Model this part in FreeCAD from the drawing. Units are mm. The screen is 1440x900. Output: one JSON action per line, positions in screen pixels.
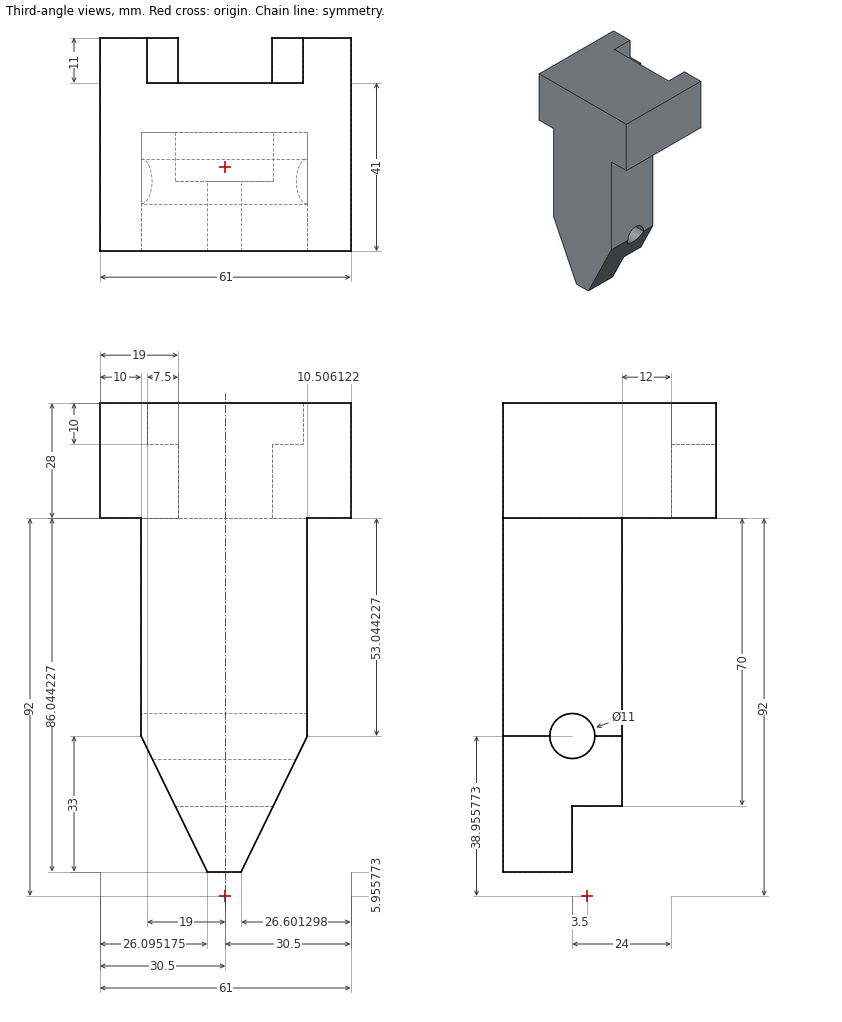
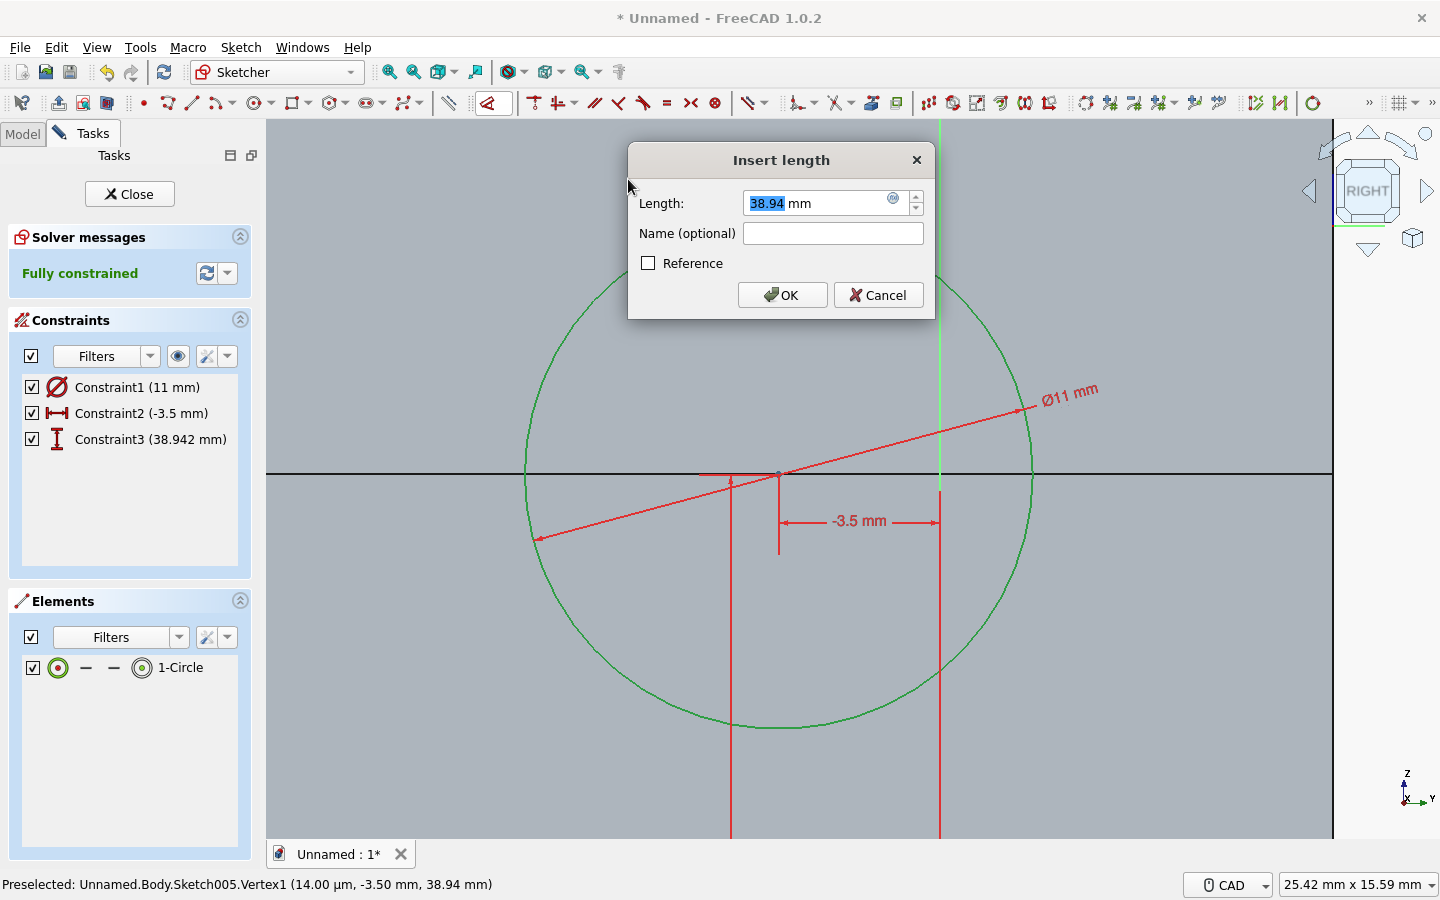
{"action": "type", "text": "38.955773"}
{"action": "key", "text": "Return"}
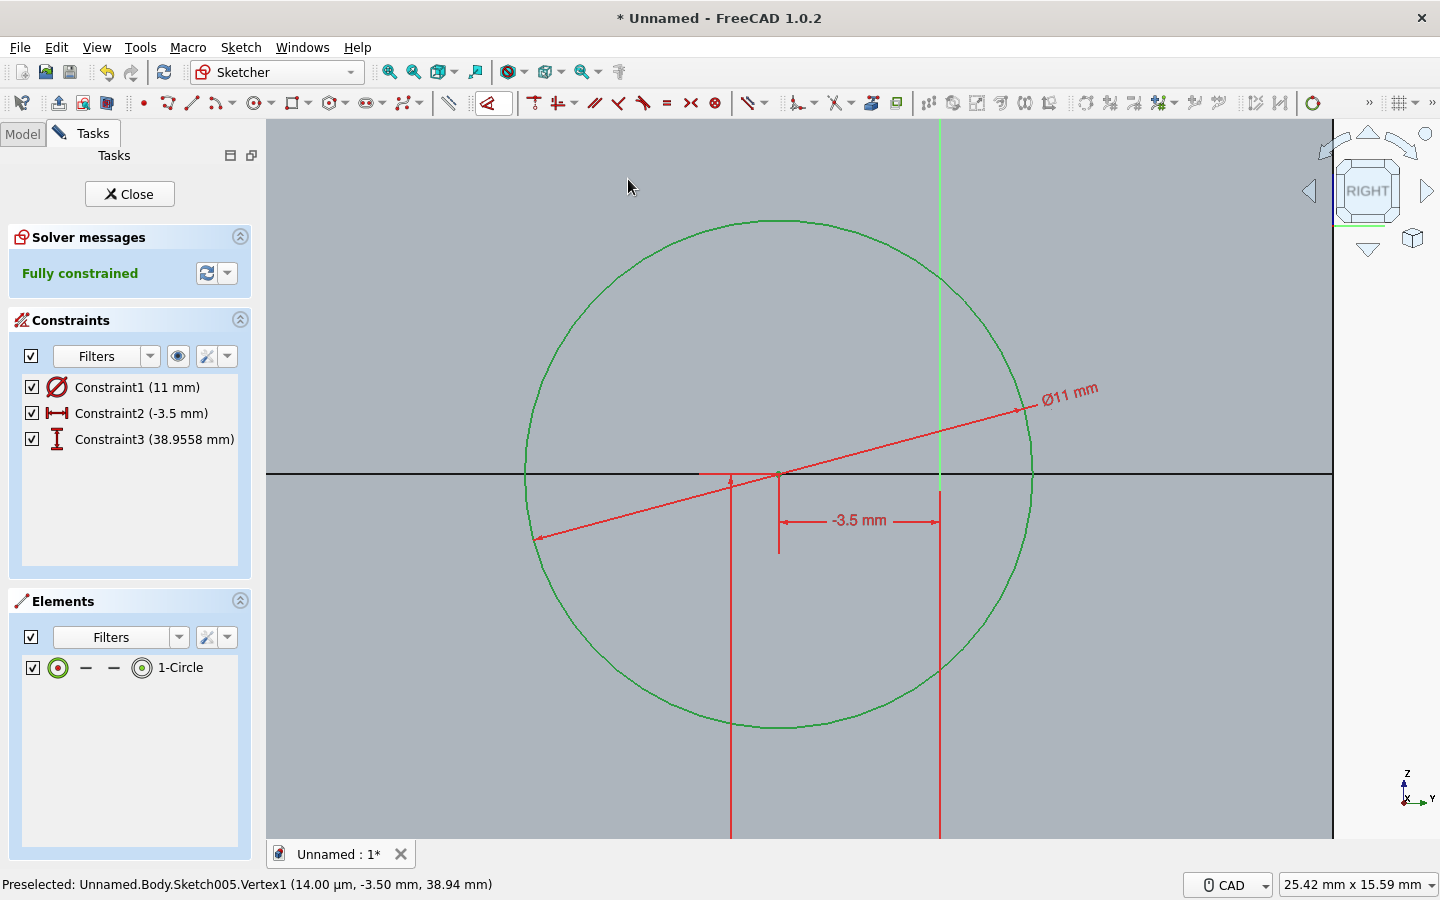
{"action": "left_click", "coordinate": [130, 194]}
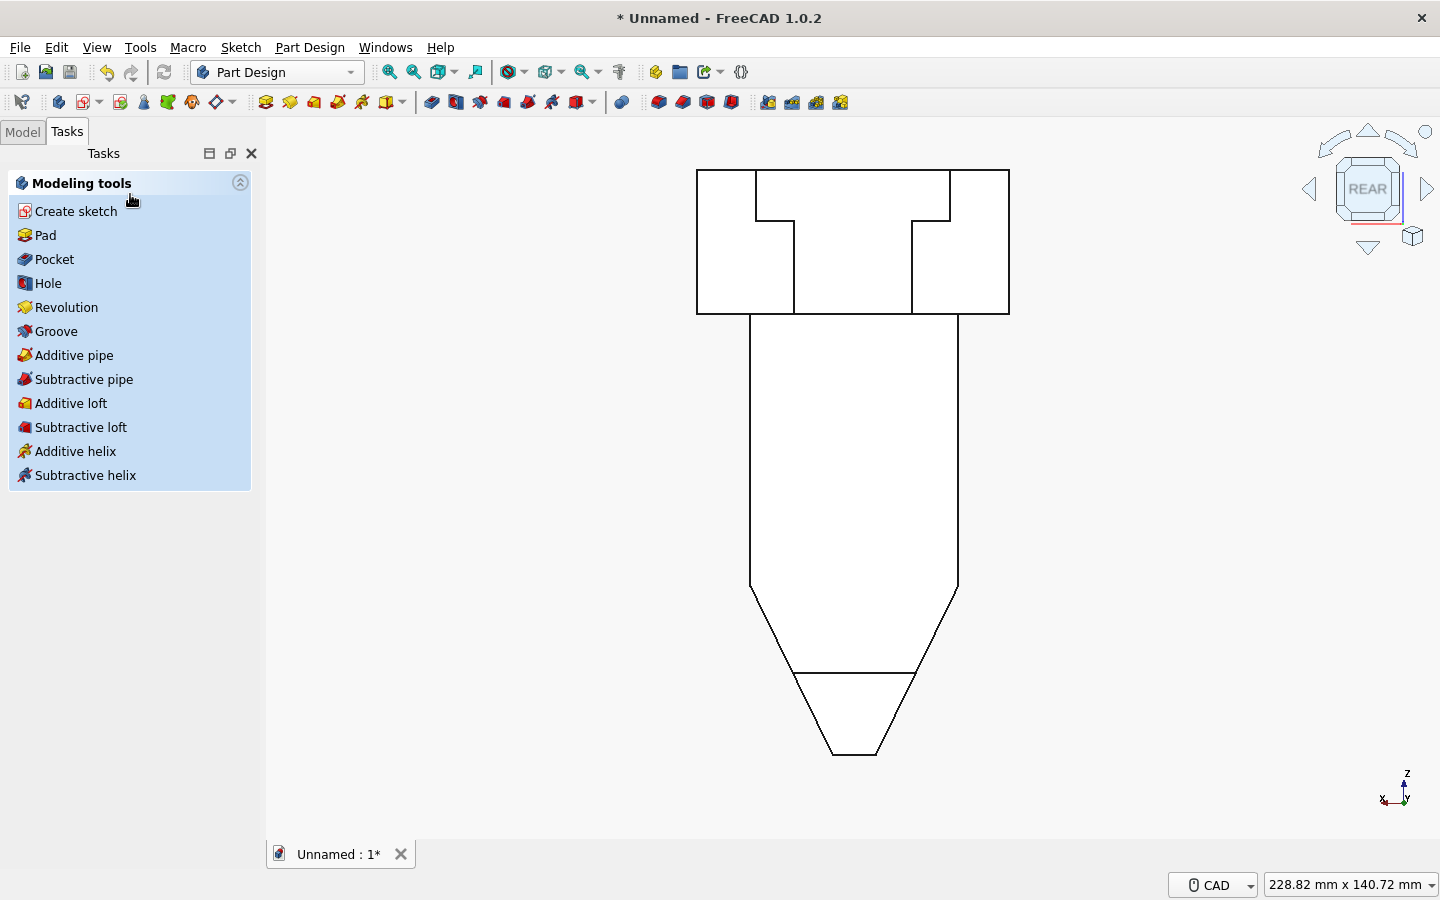
{"action": "left_click", "coordinate": [432, 102]}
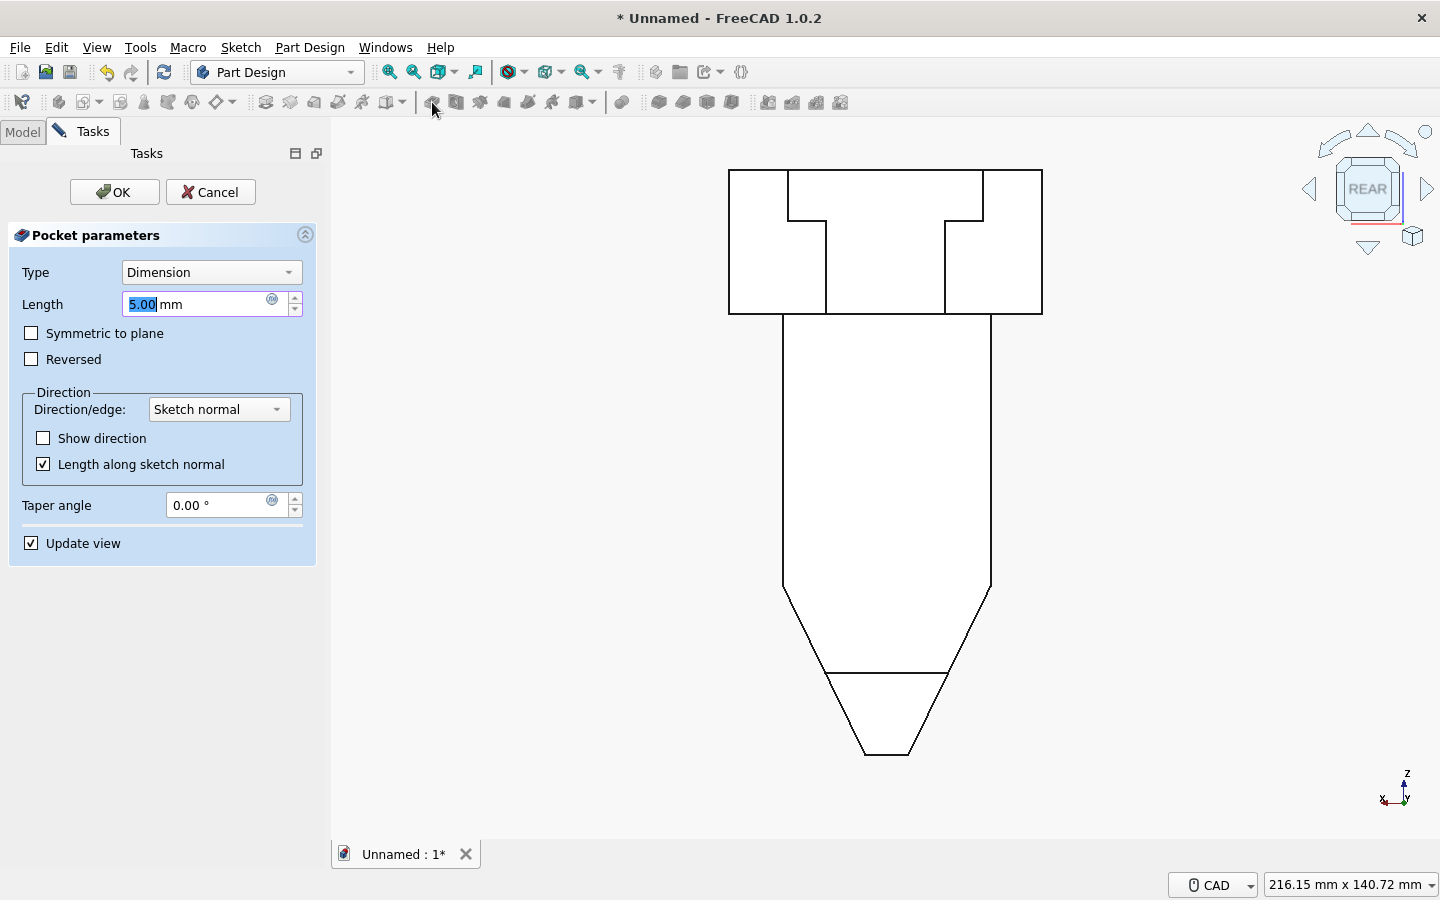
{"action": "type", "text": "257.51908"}
{"action": "key", "text": "Tab"}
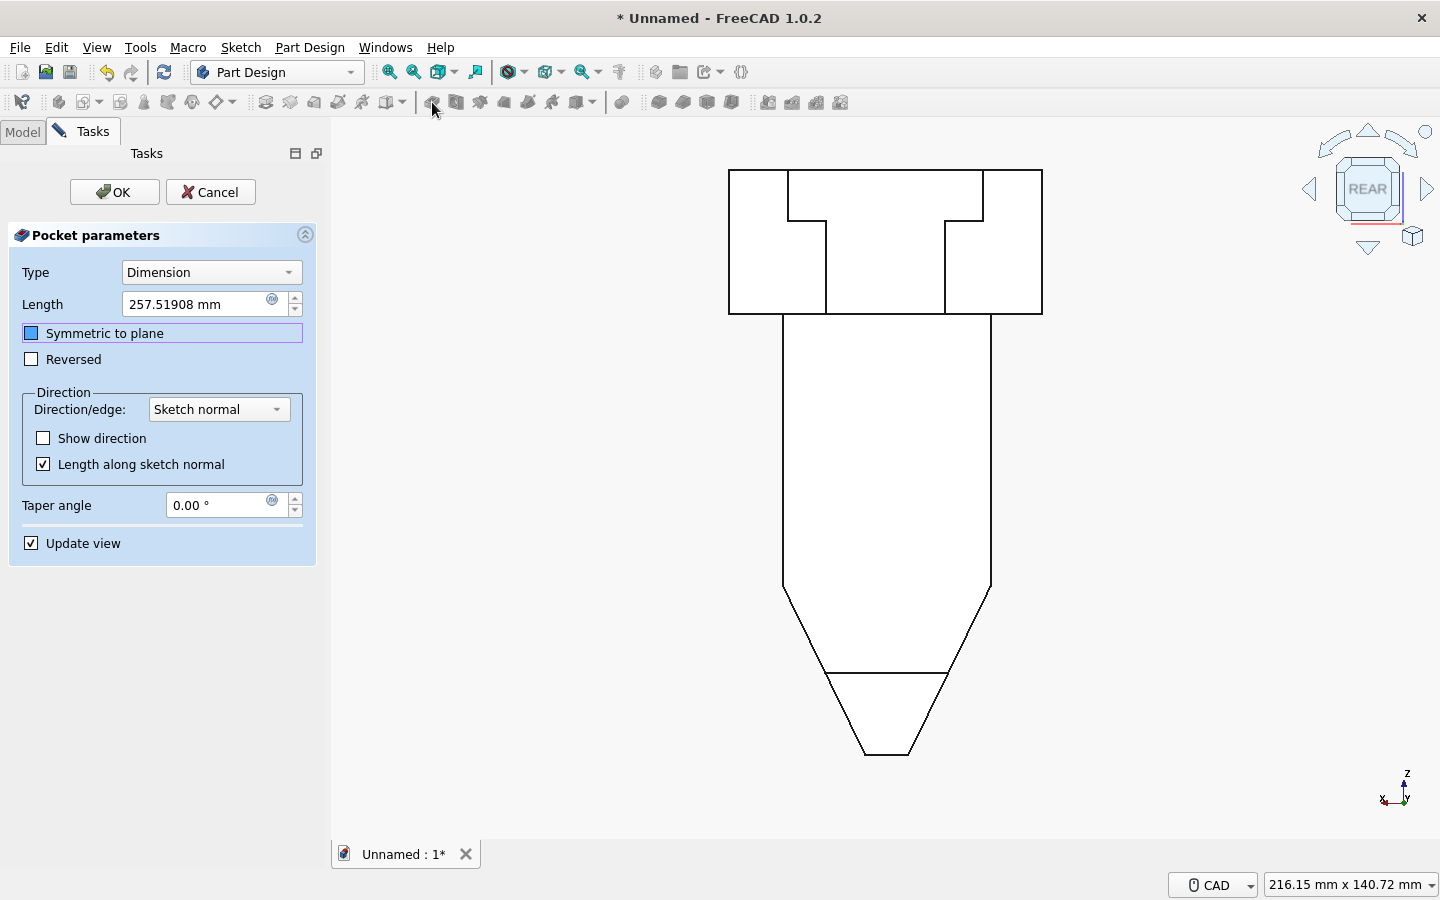
{"action": "left_click", "coordinate": [30, 333]}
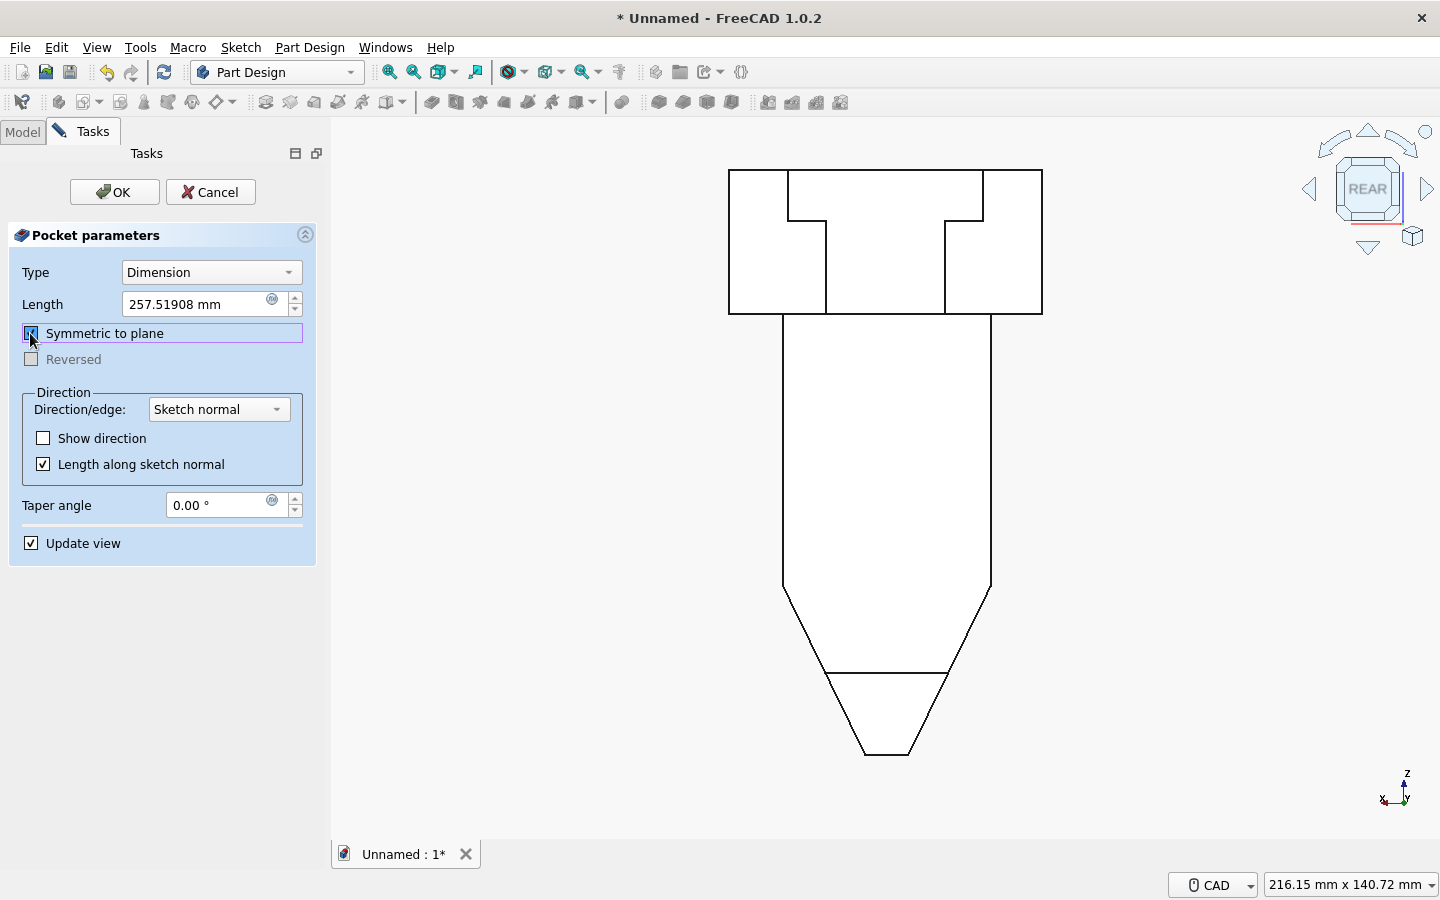
{"action": "left_click", "coordinate": [115, 192]}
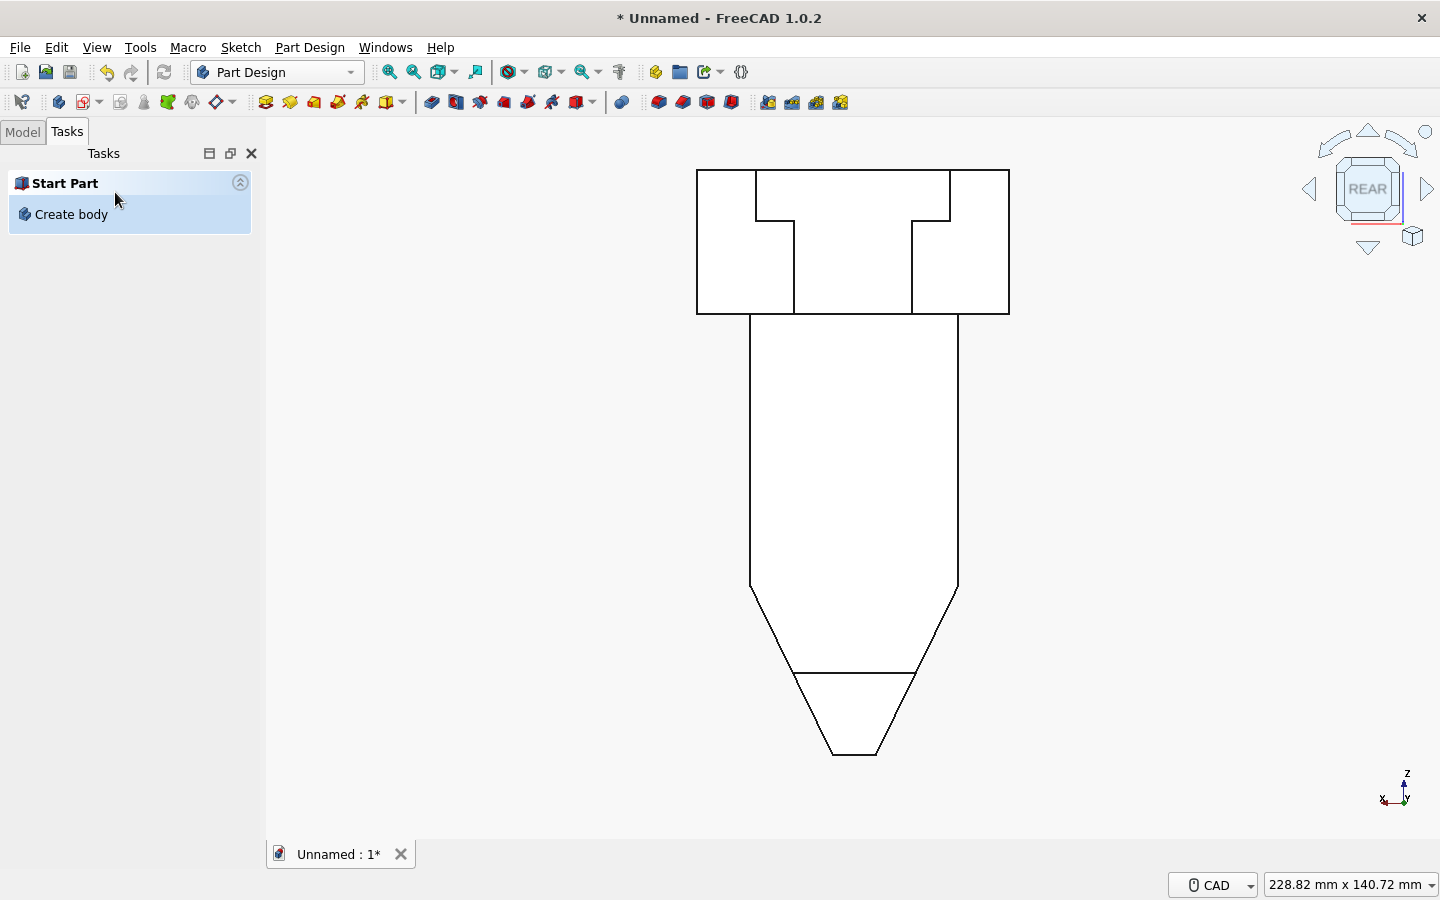
{"action": "key", "text": "0"}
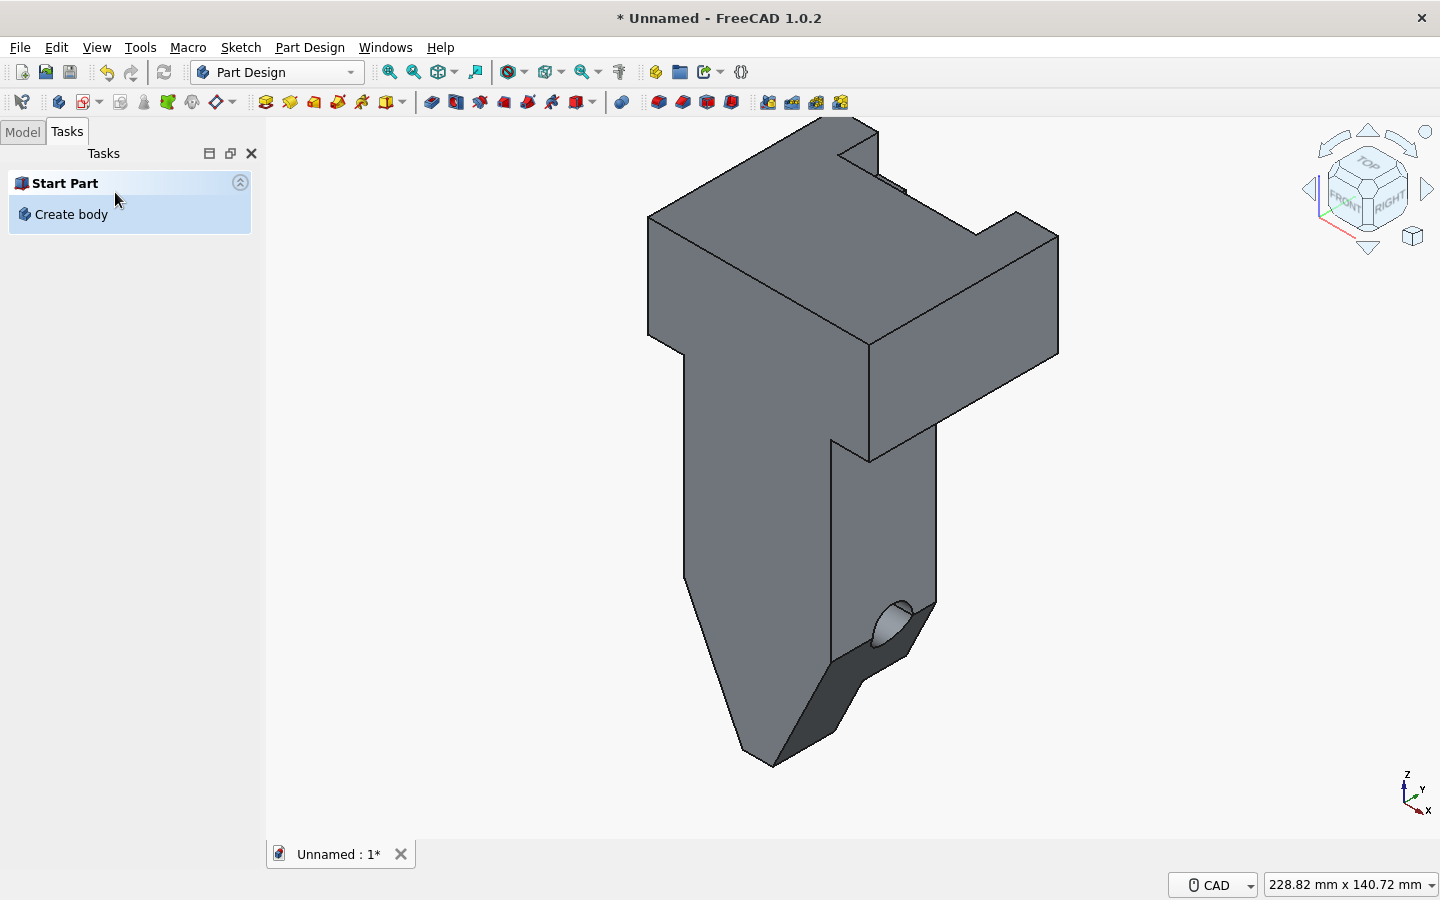
{"action": "left_click", "coordinate": [390, 72]}